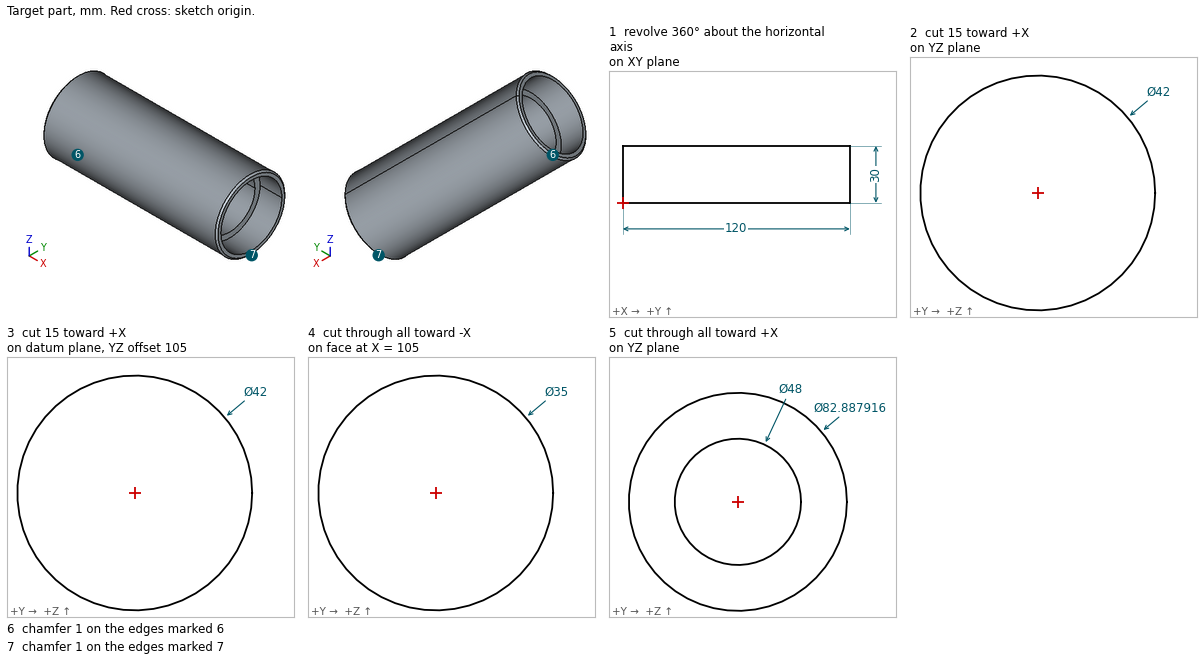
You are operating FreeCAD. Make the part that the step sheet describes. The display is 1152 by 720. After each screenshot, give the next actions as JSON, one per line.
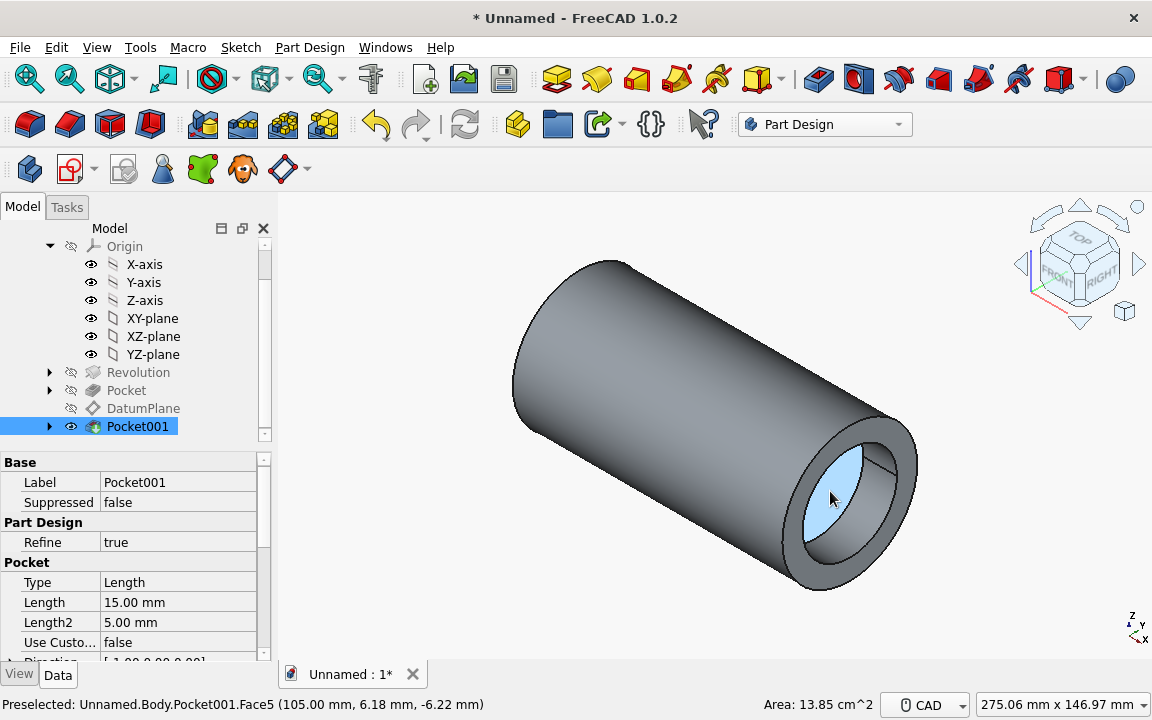
{"action": "left_click", "coordinate": [70, 170]}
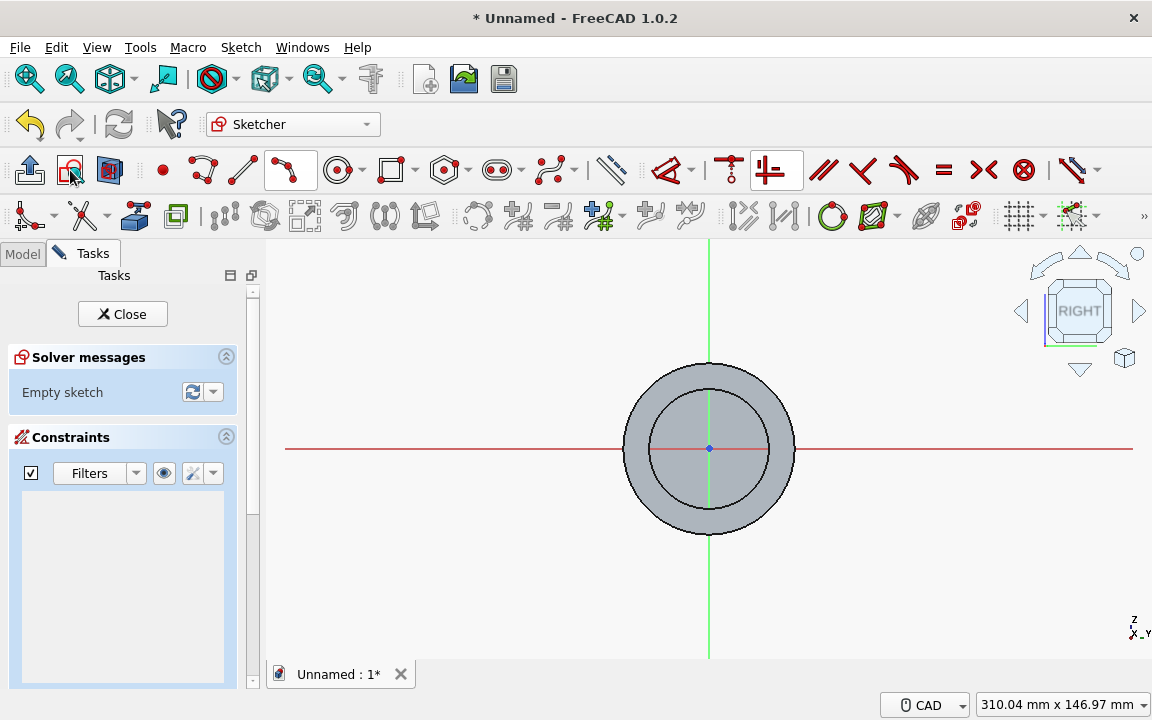
{"action": "scroll", "coordinate": [749, 449], "scroll_direction": "up", "scroll_amount": 5}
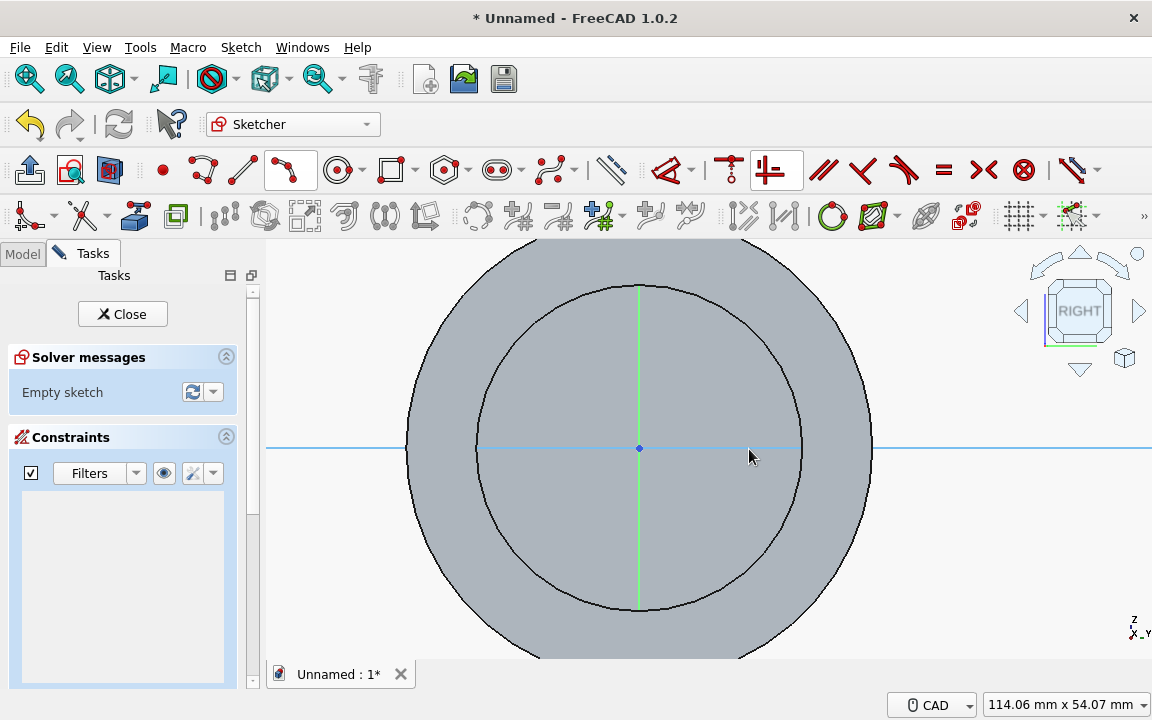
{"action": "left_click", "coordinate": [338, 170]}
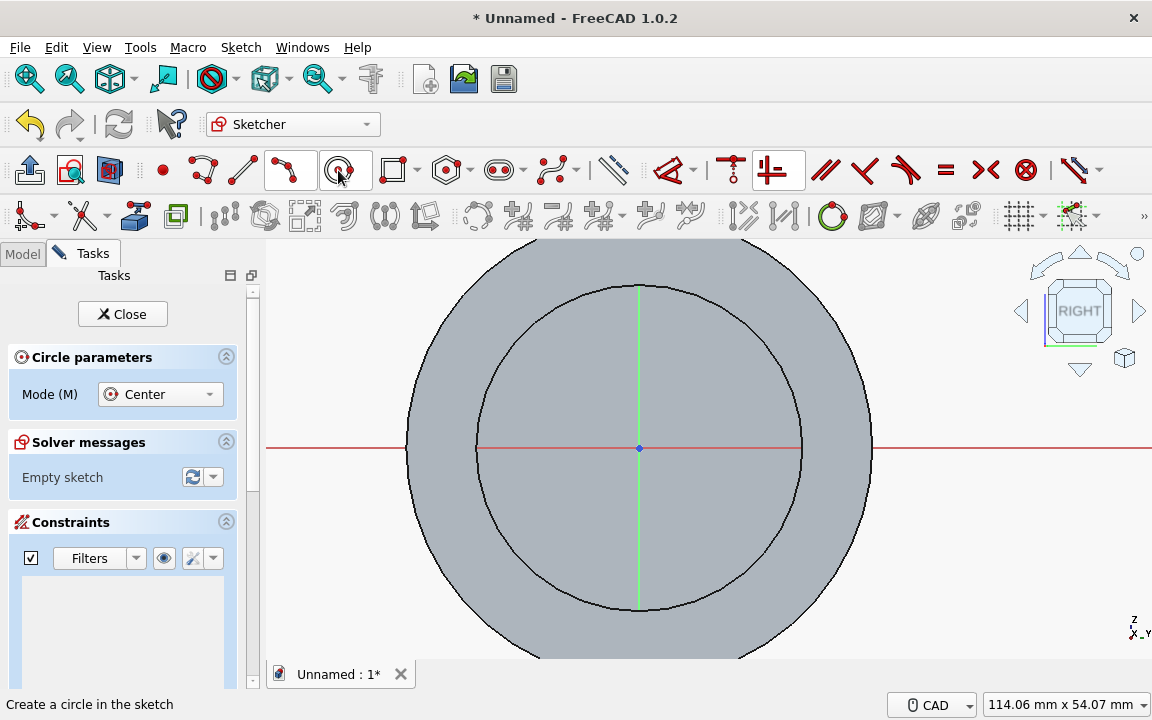
{"action": "left_click", "coordinate": [639, 448]}
{"action": "left_click", "coordinate": [735, 352]}
{"action": "key", "text": "Escape"}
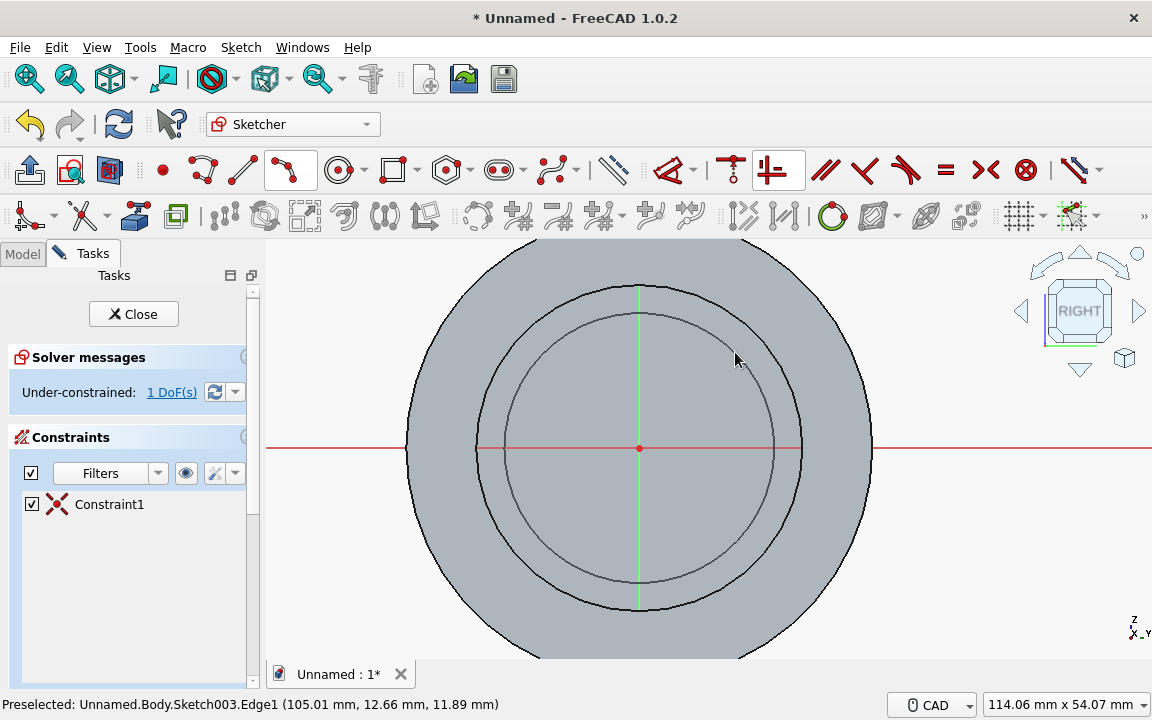
{"action": "key", "text": "d"}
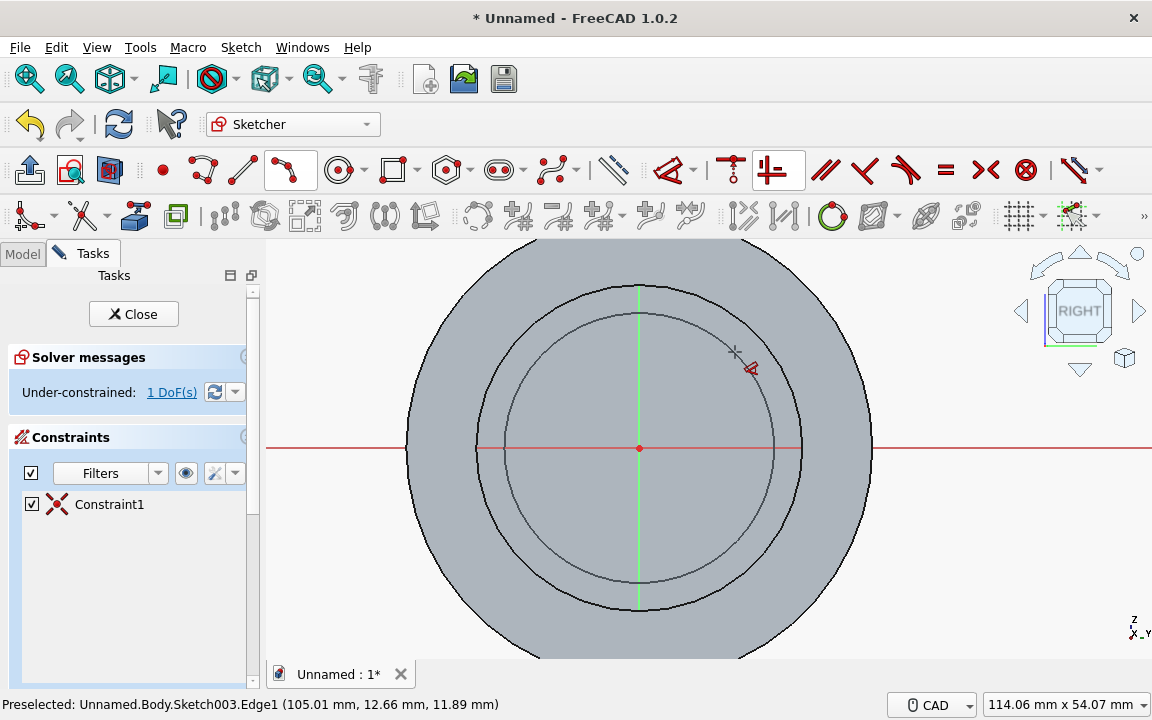
{"action": "left_click", "coordinate": [734, 352]}
{"action": "left_click", "coordinate": [756, 329]}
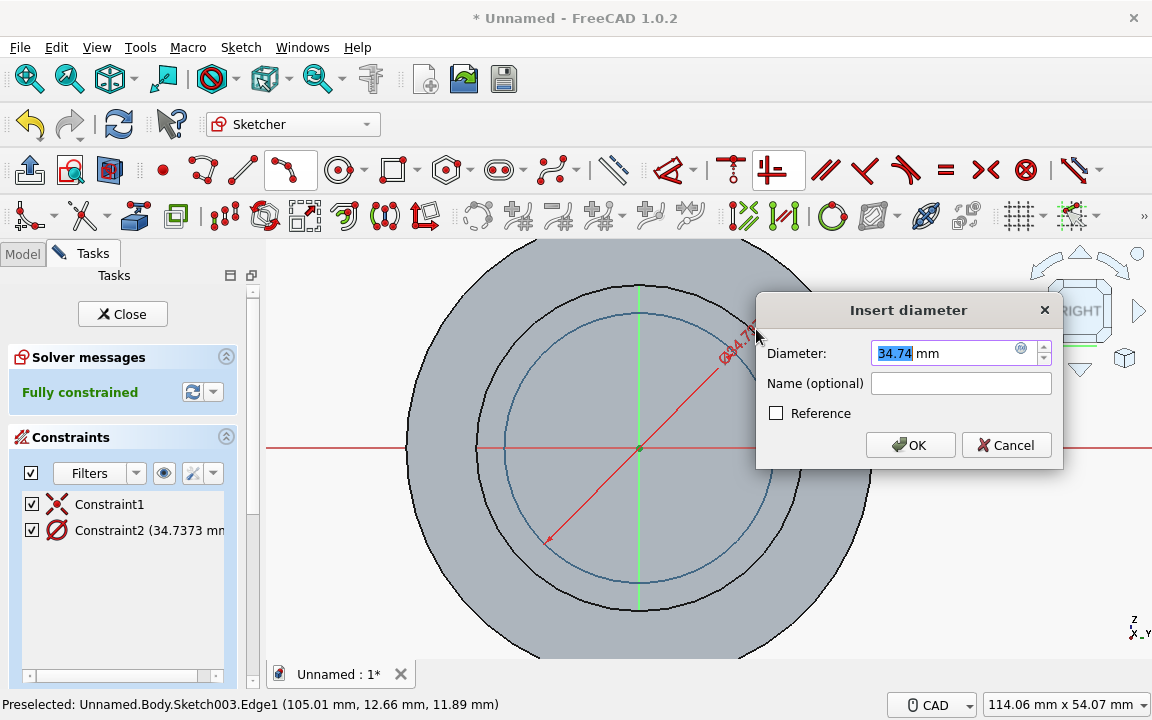
{"action": "type", "text": "35"}
{"action": "key", "text": "Return"}
{"action": "key", "text": "Escape"}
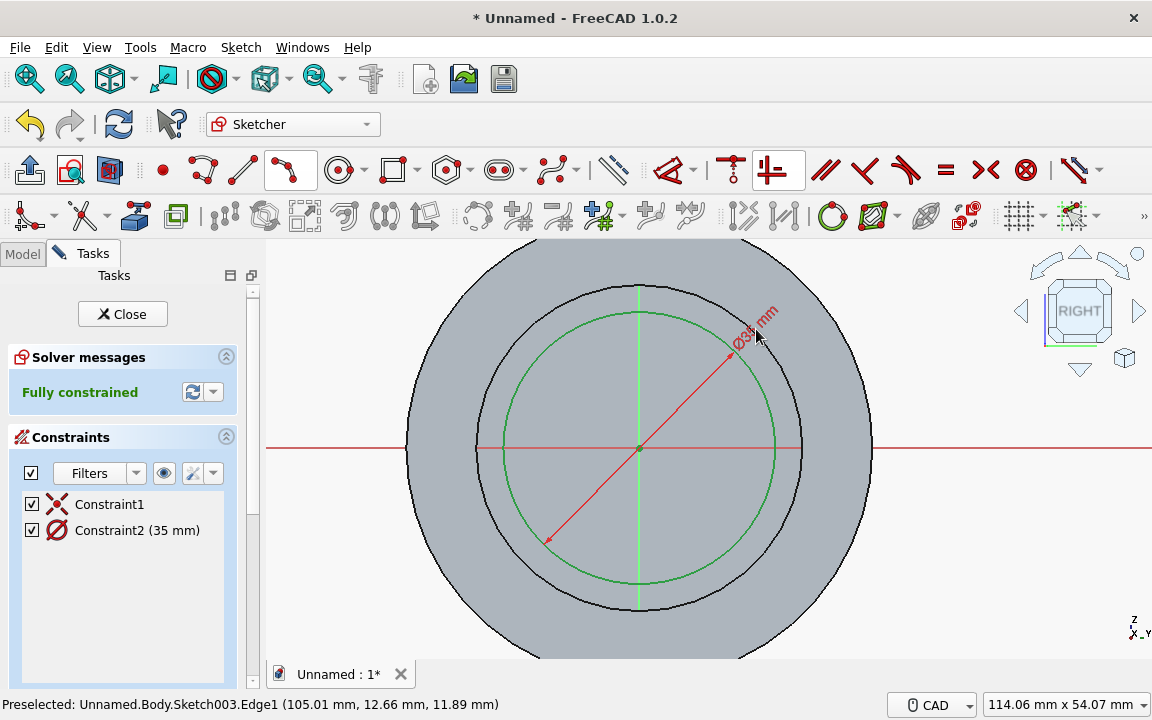
{"action": "left_click", "coordinate": [123, 314]}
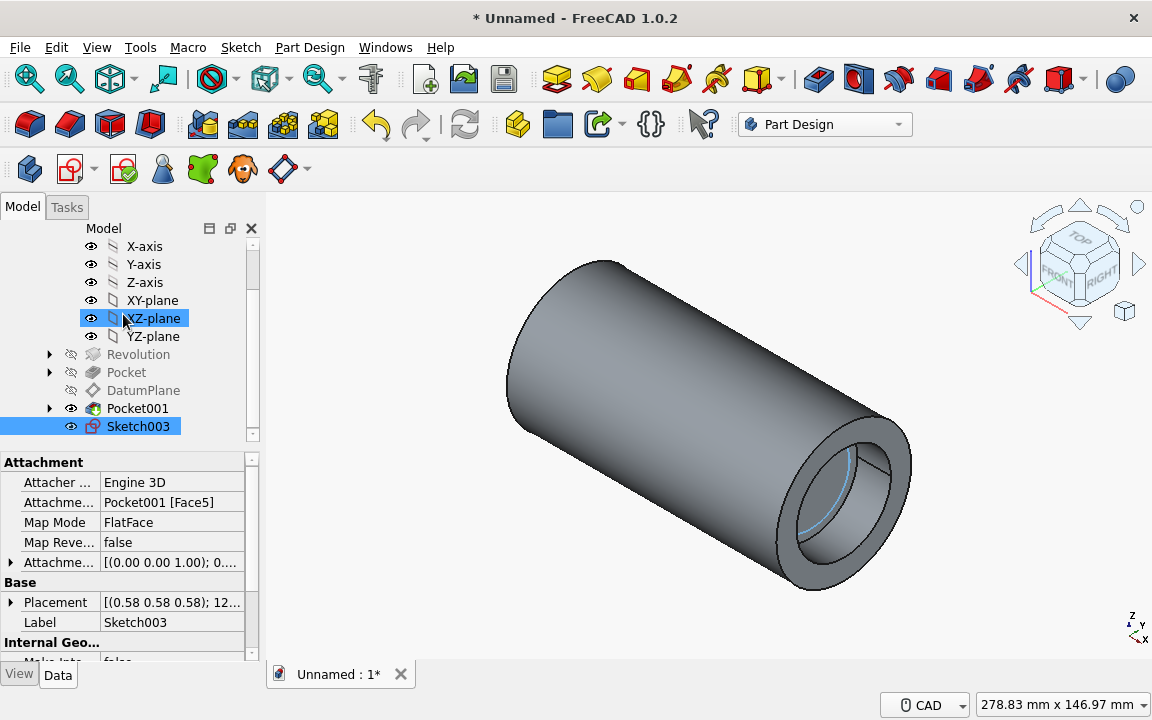
{"action": "left_click", "coordinate": [820, 80]}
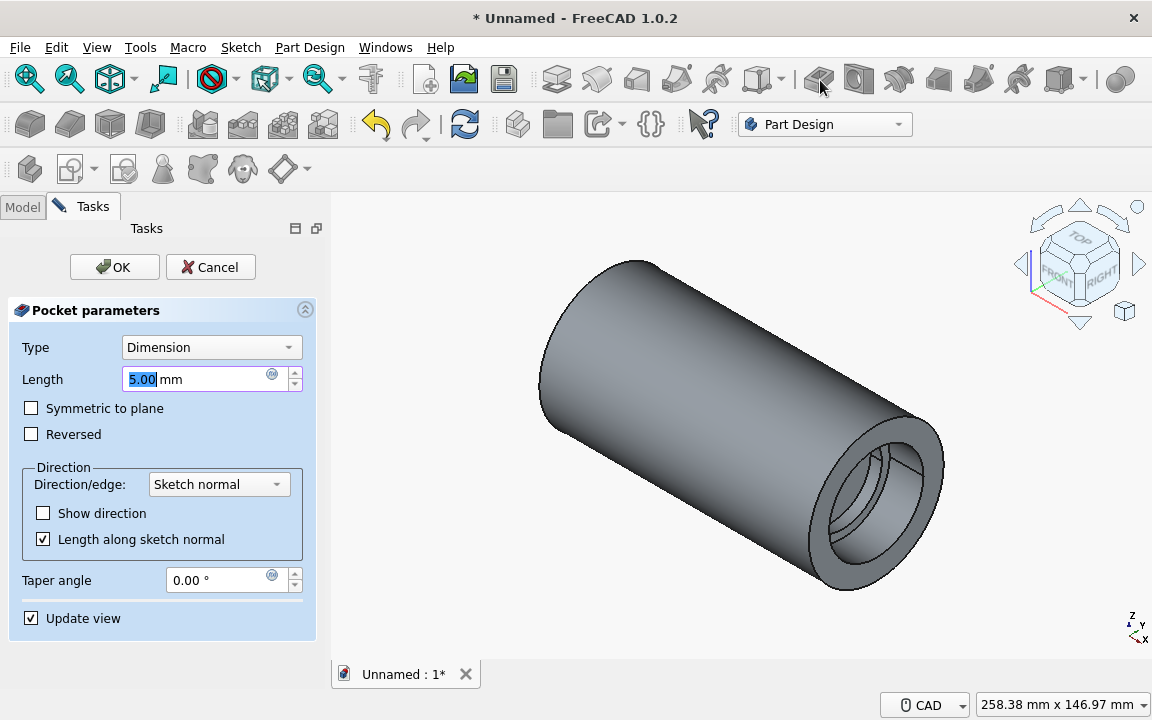
{"action": "left_click", "coordinate": [212, 348]}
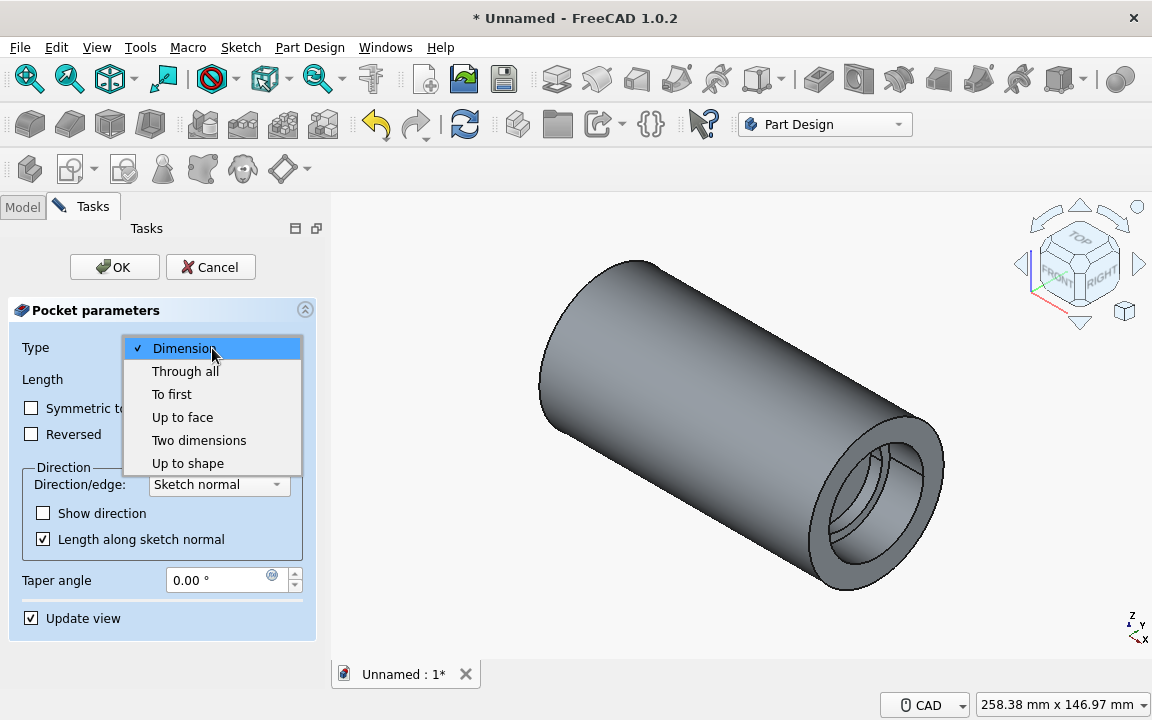
{"action": "left_click", "coordinate": [212, 372]}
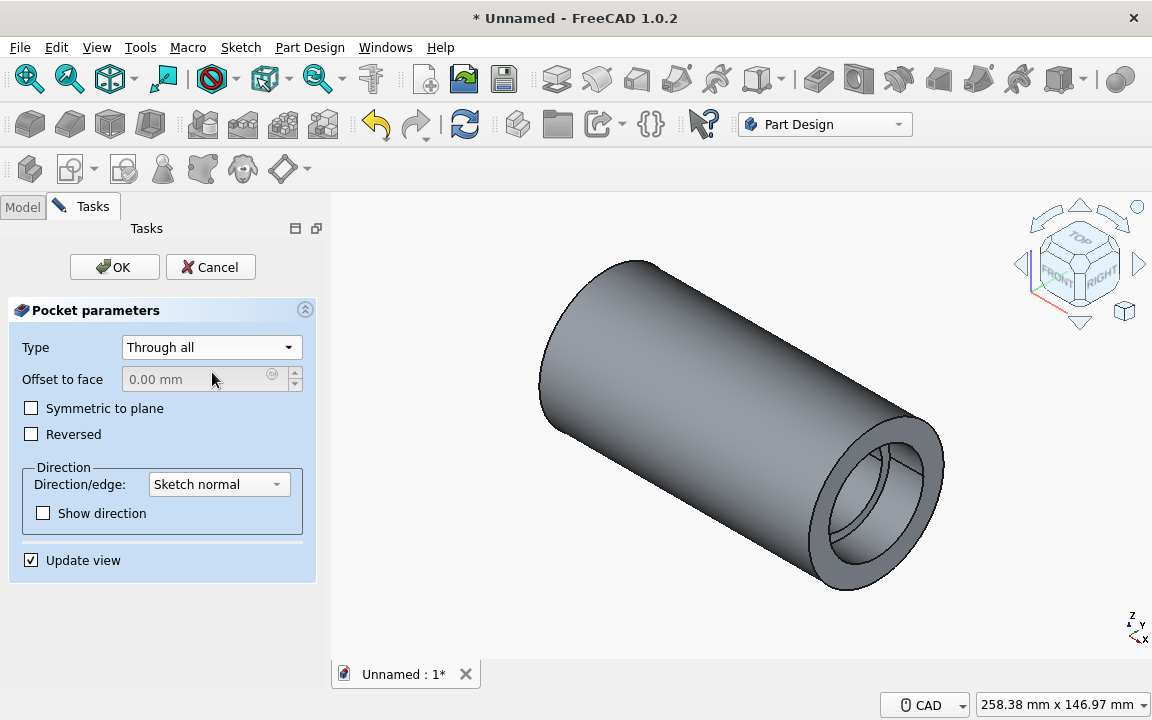
{"action": "left_click", "coordinate": [115, 267]}